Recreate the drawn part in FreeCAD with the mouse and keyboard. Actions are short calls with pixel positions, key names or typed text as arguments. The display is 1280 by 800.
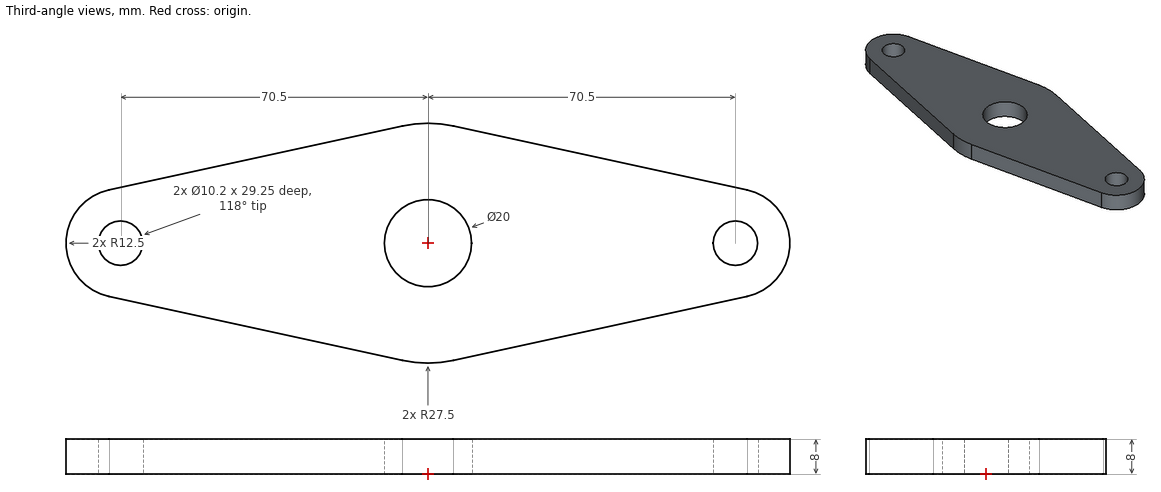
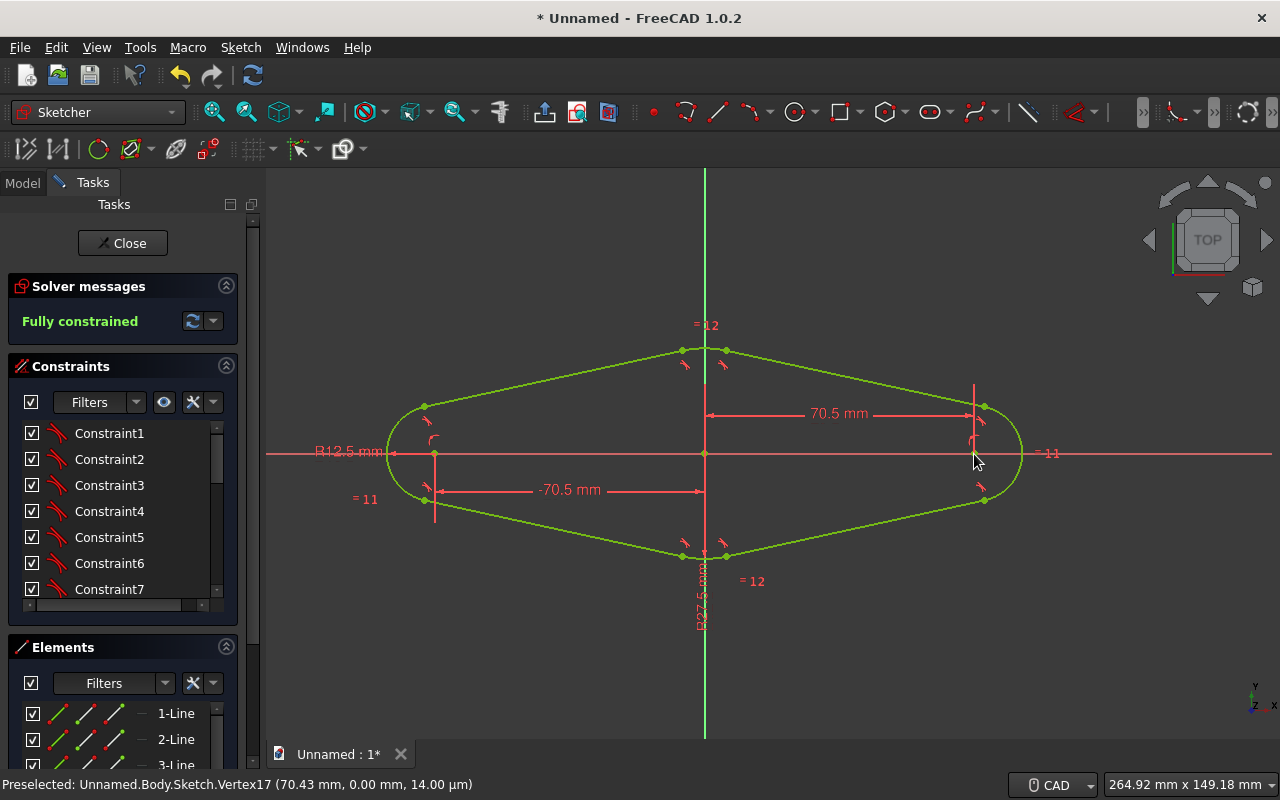
click(123, 243)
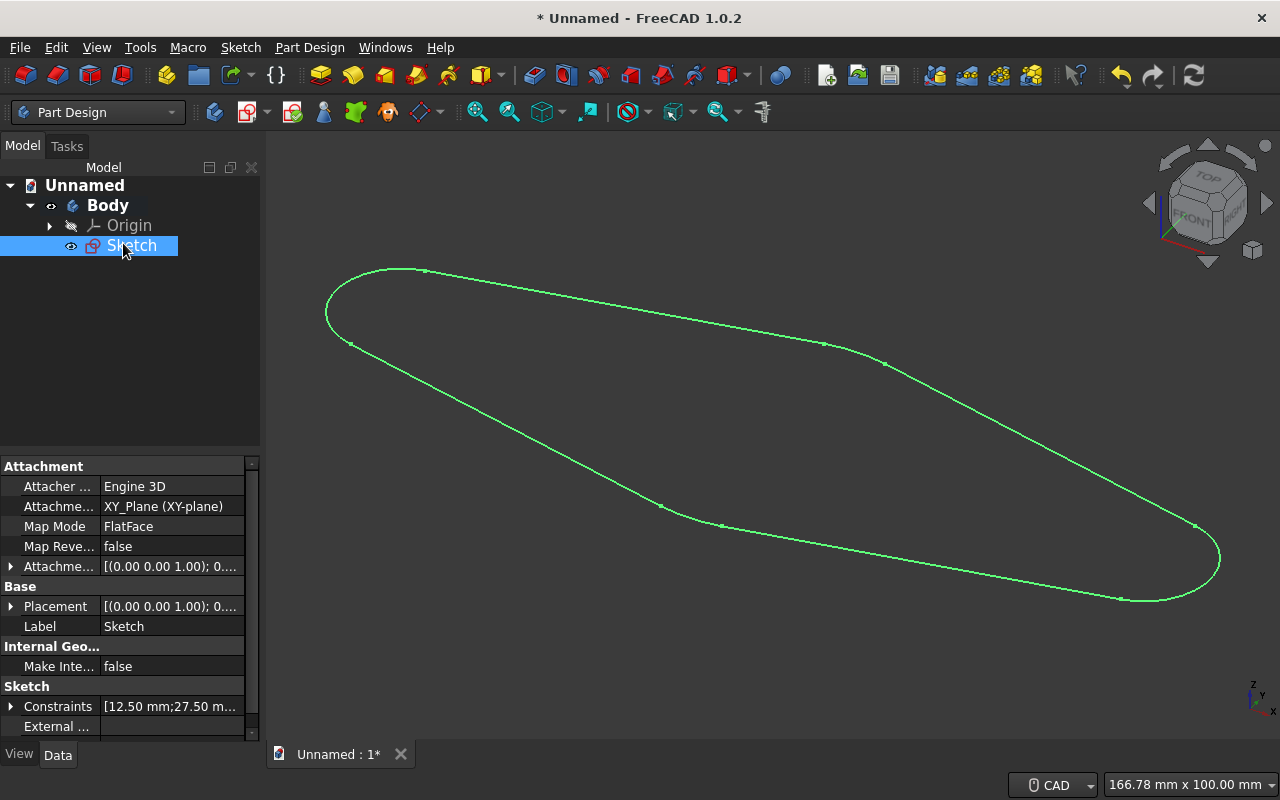
click(322, 76)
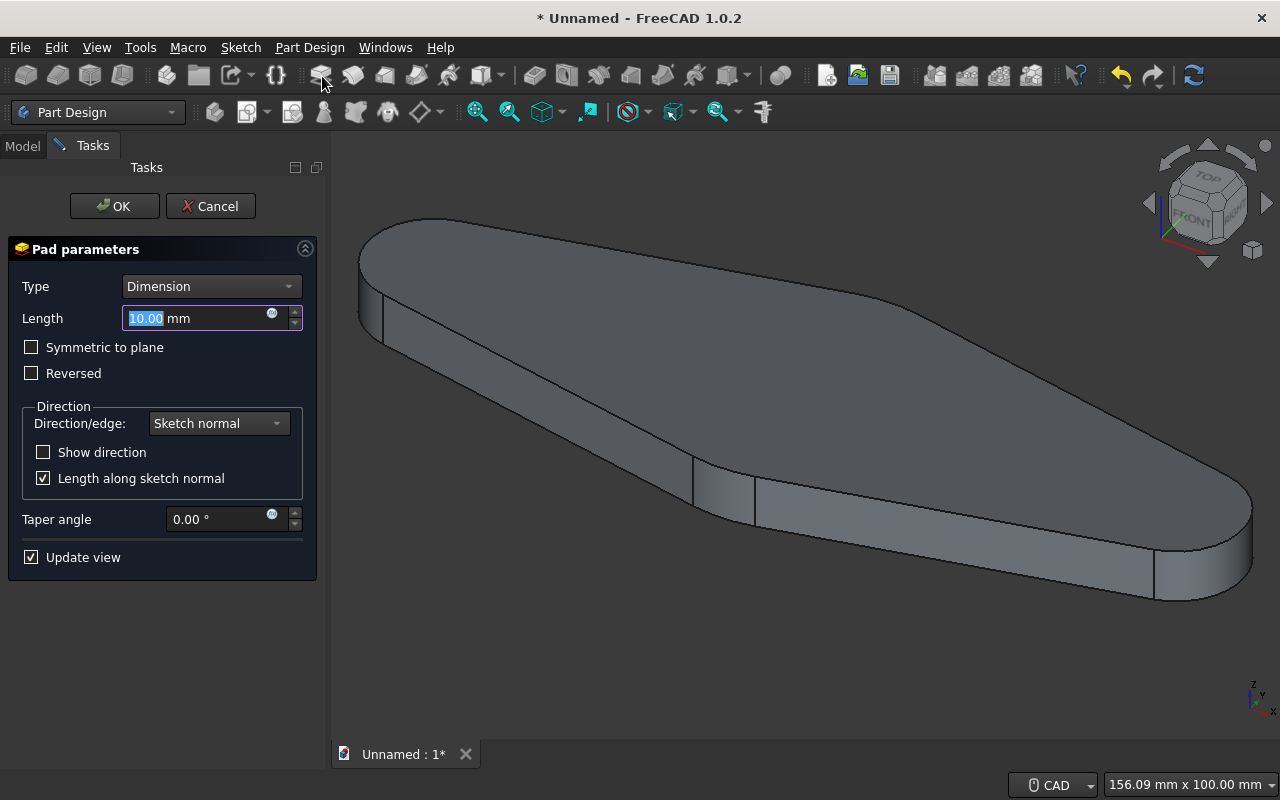
text(8)
key(Tab)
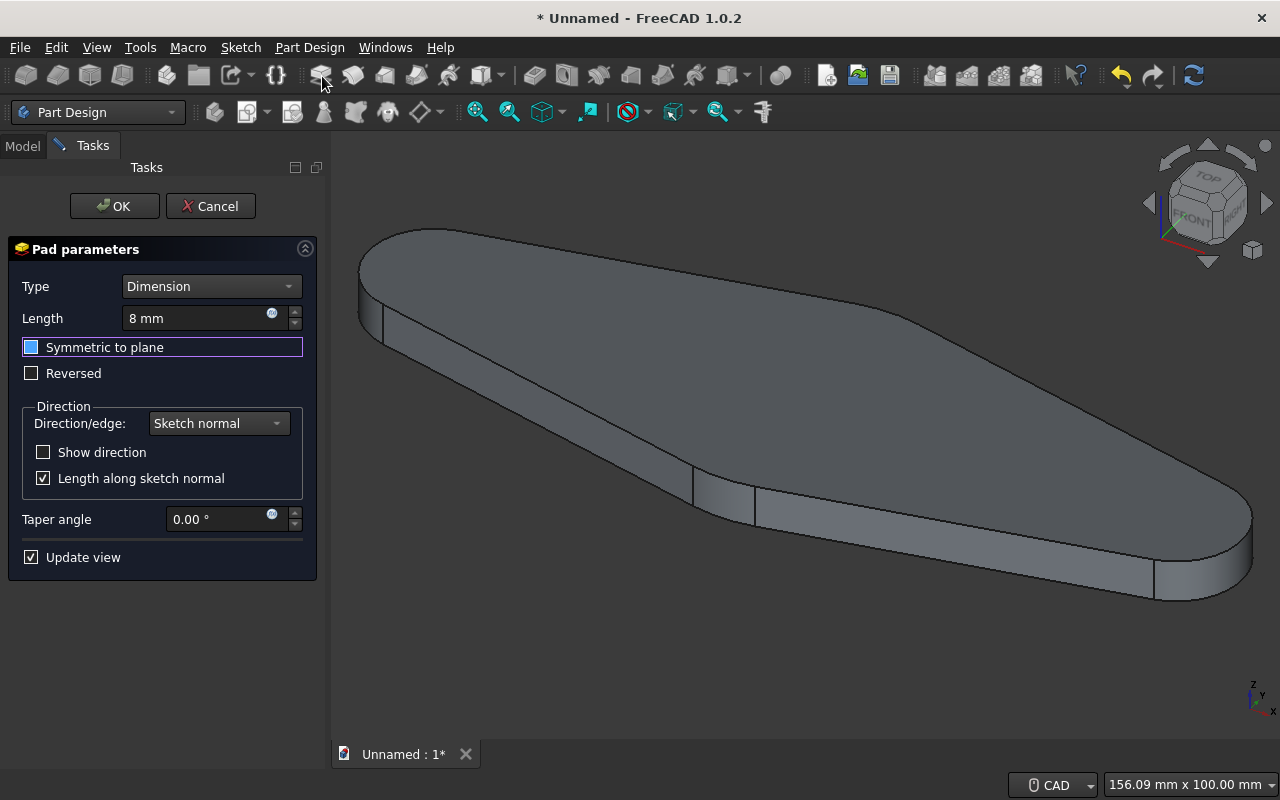
click(115, 206)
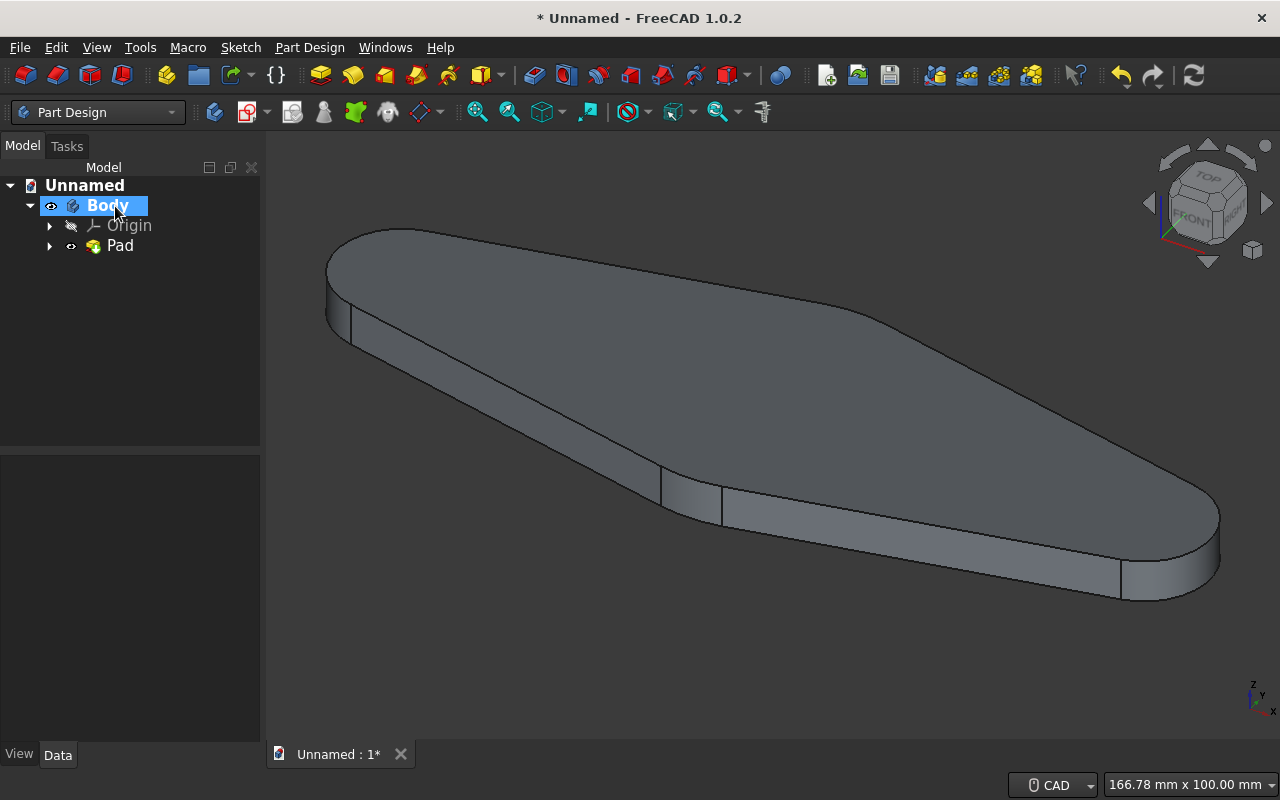
click(478, 112)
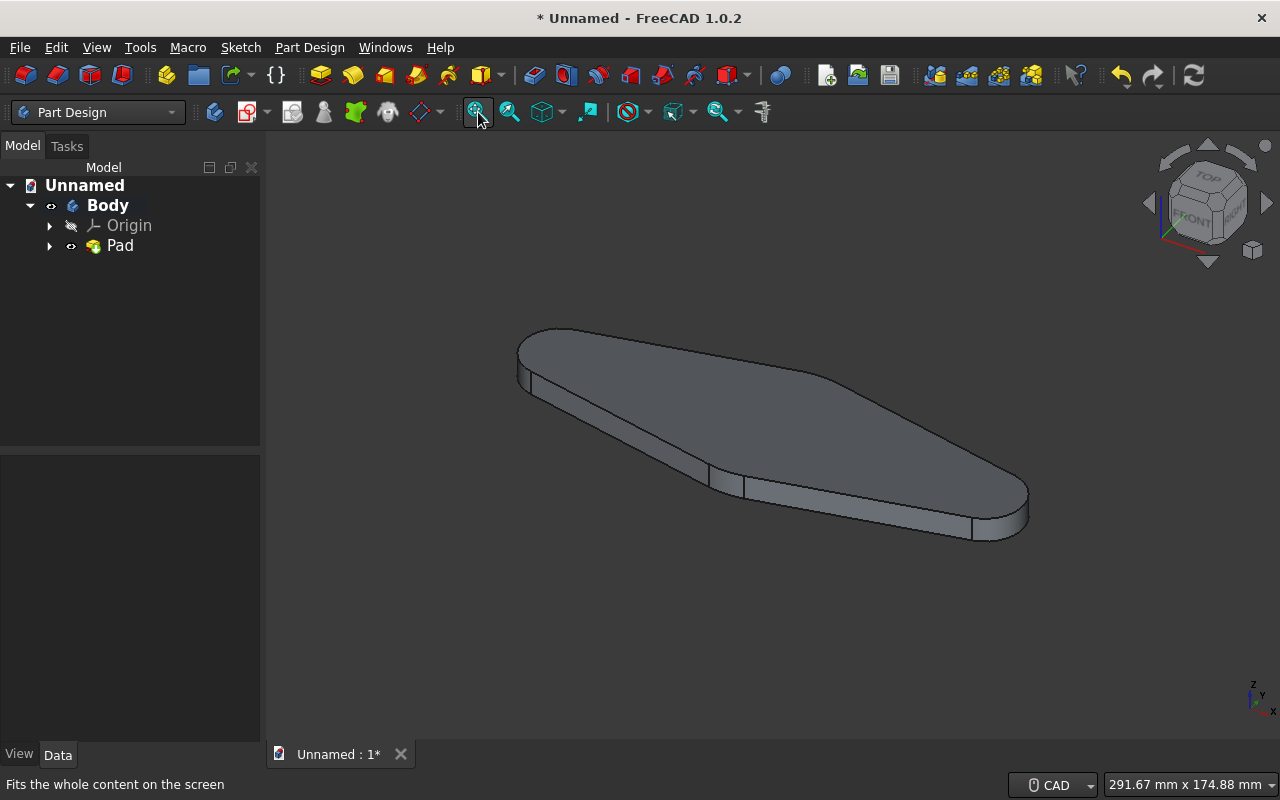
click(773, 423)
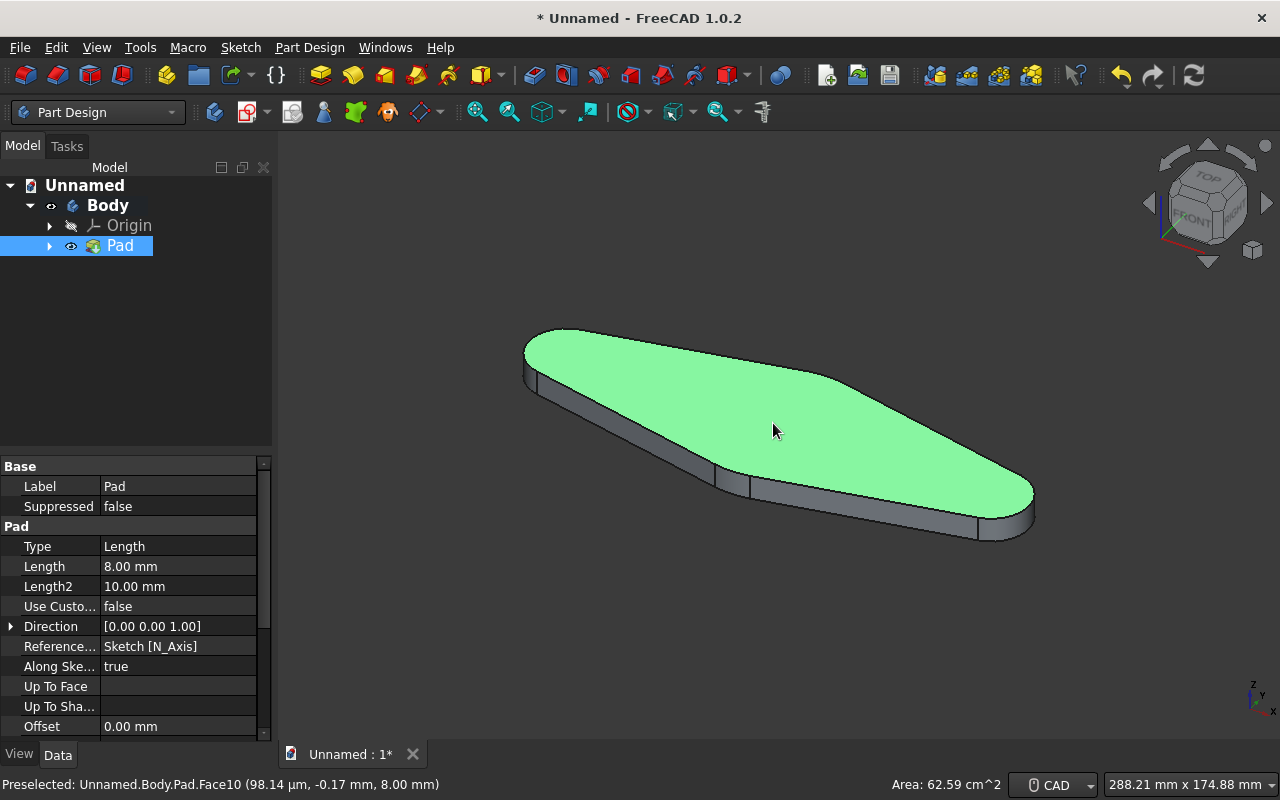
click(248, 112)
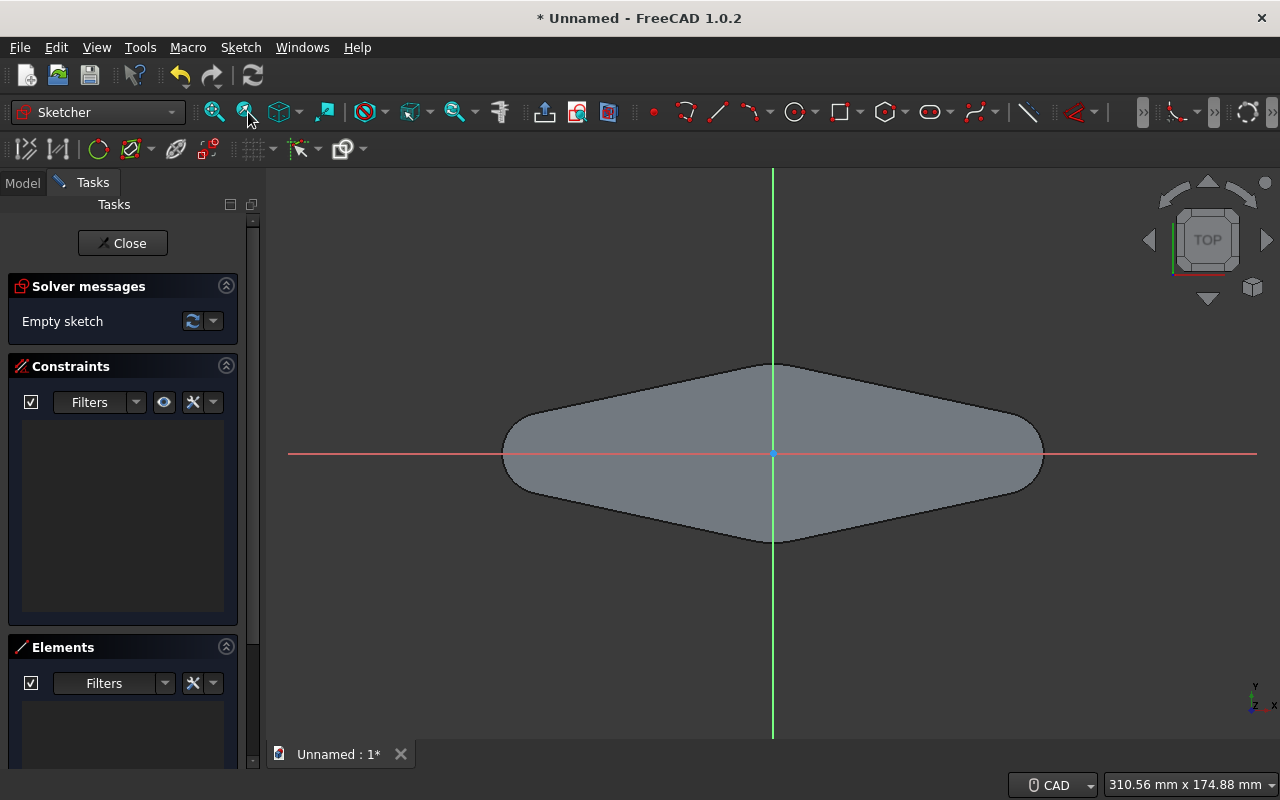
click(796, 112)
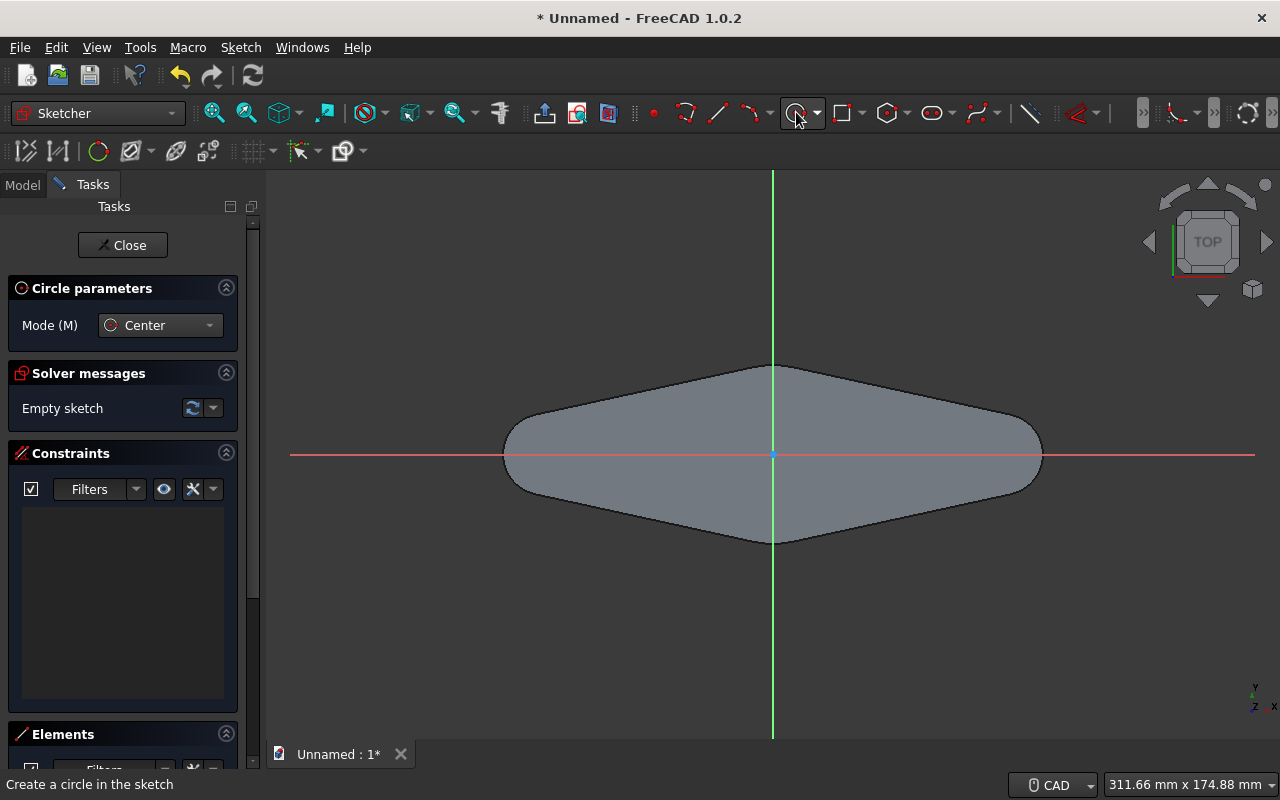
scroll(544, 454, up, 2)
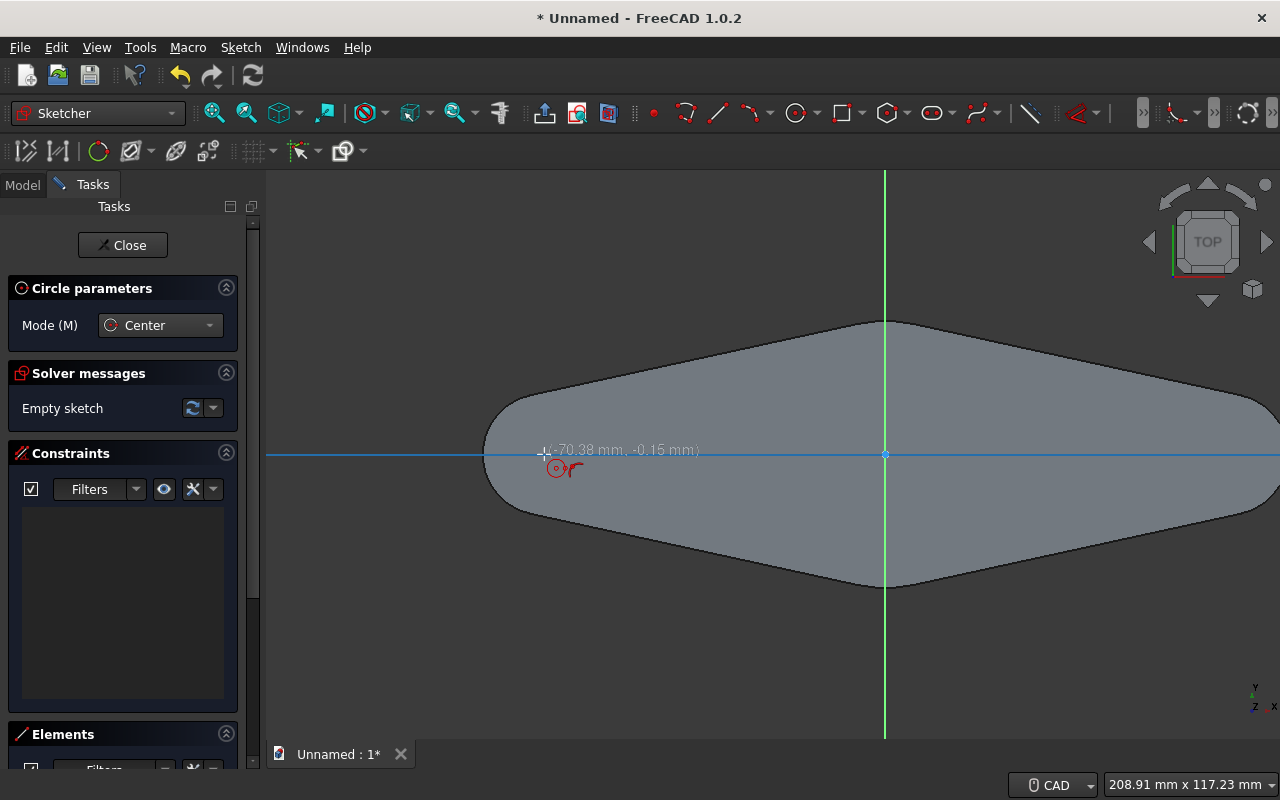
click(543, 454)
move(561, 437)